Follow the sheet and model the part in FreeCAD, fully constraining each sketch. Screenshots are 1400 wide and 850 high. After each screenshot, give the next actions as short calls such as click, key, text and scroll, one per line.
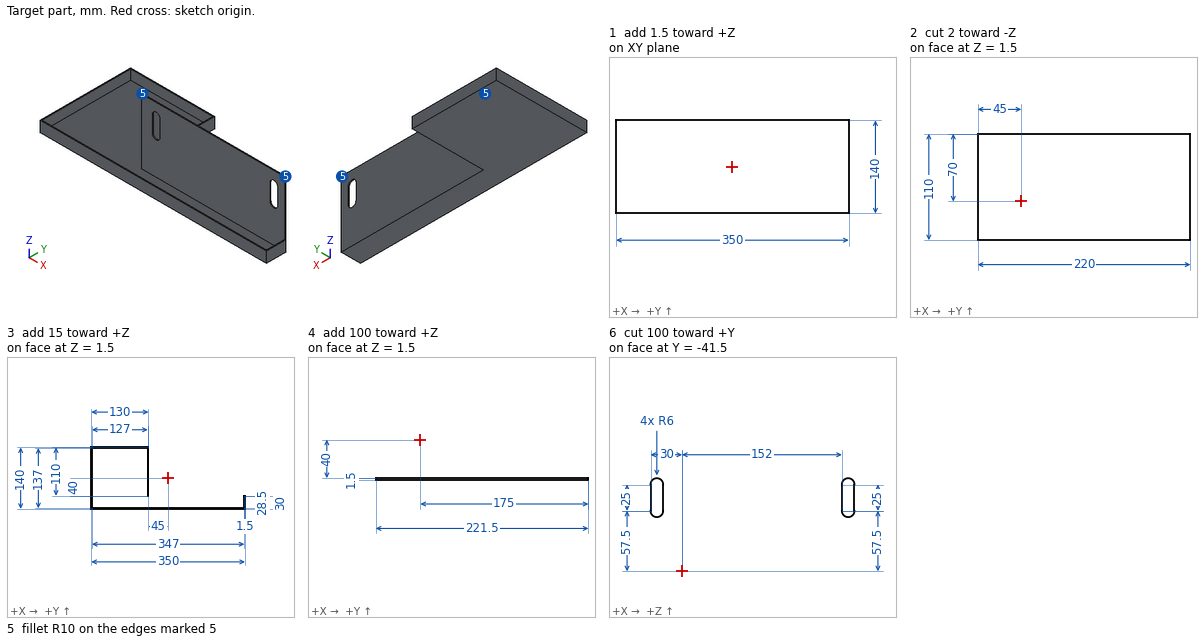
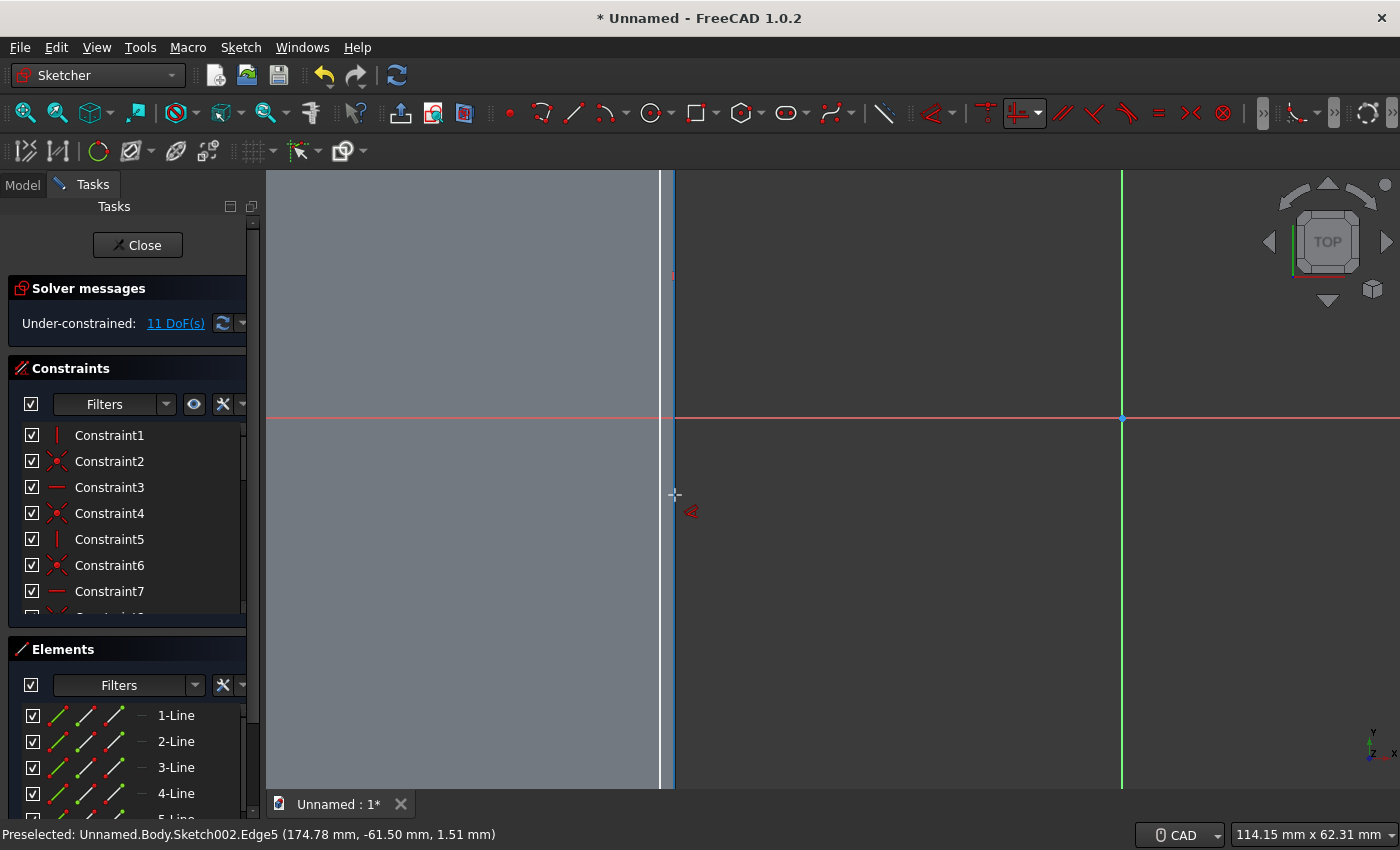
click(674, 491)
click(640, 480)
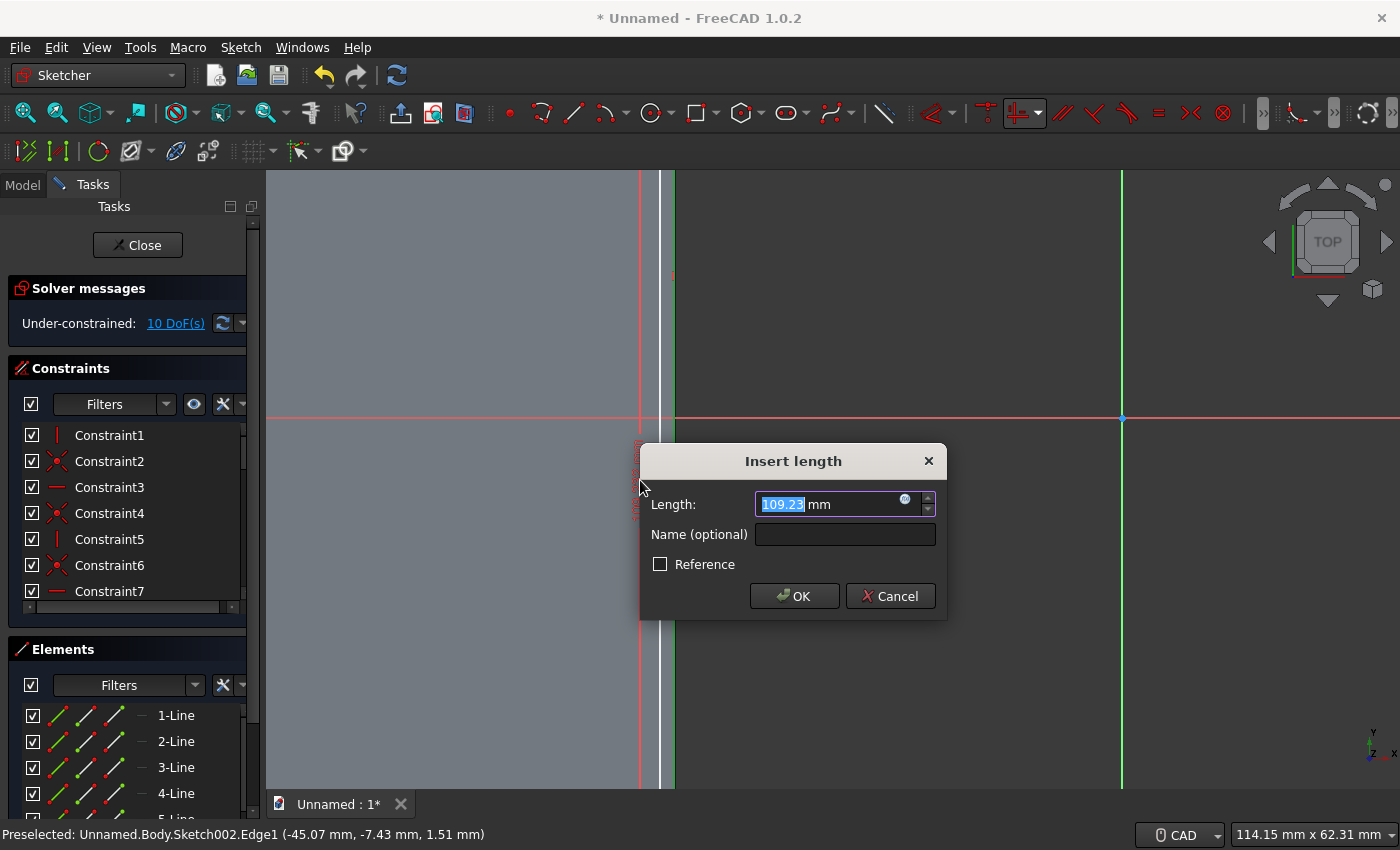
text(110)
key(Return)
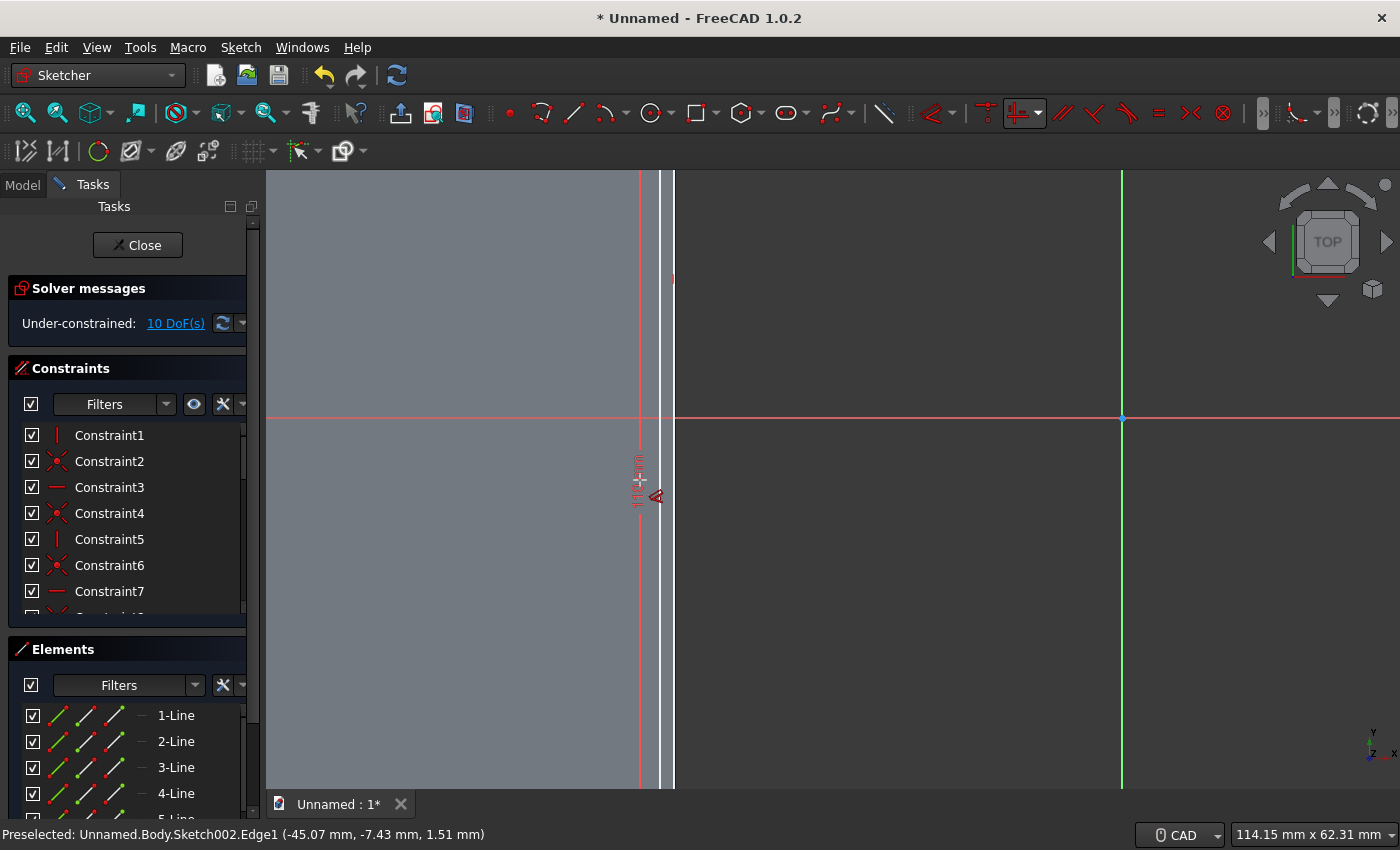
scroll(674, 495, down, 8)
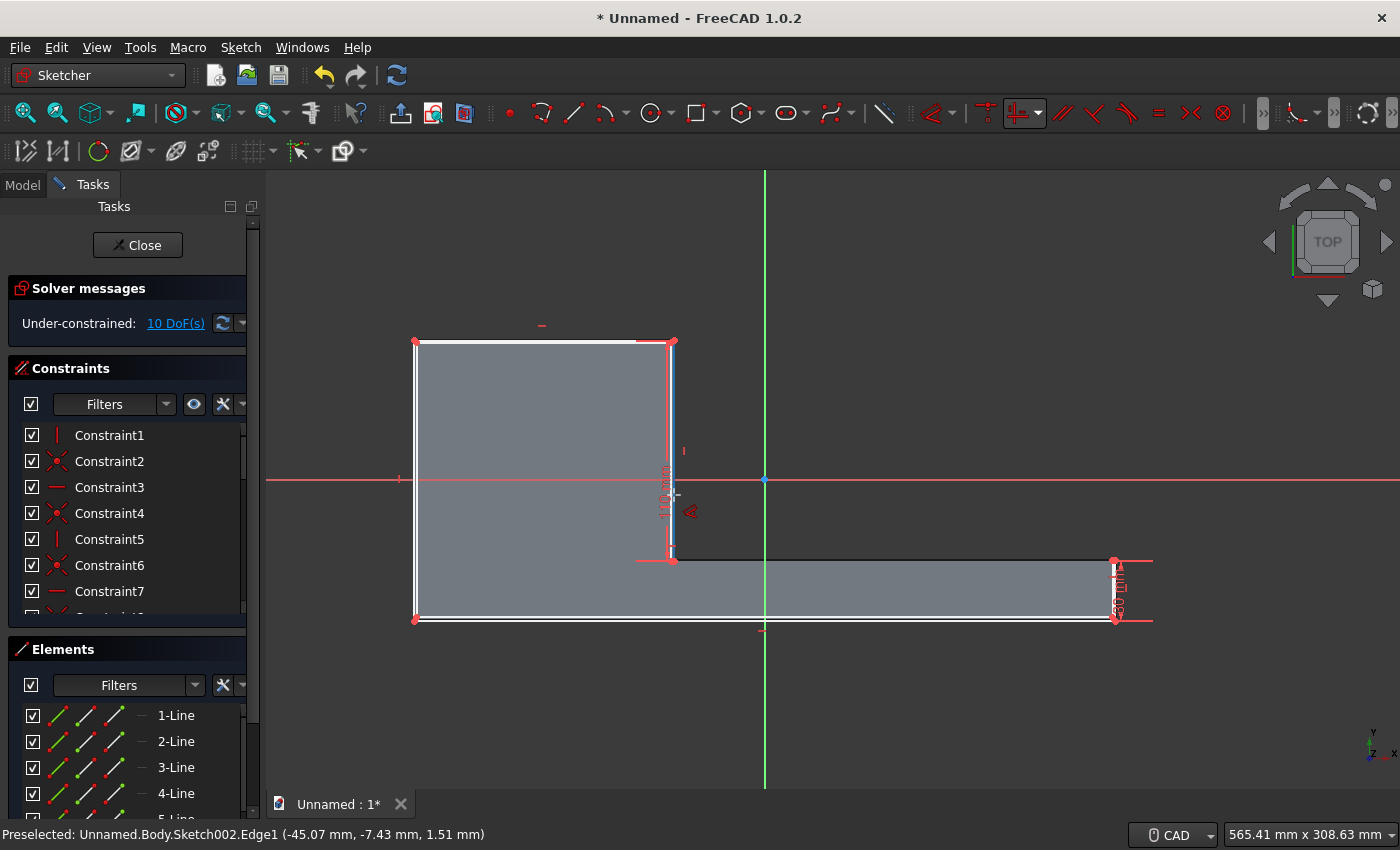
scroll(596, 341, up, 10)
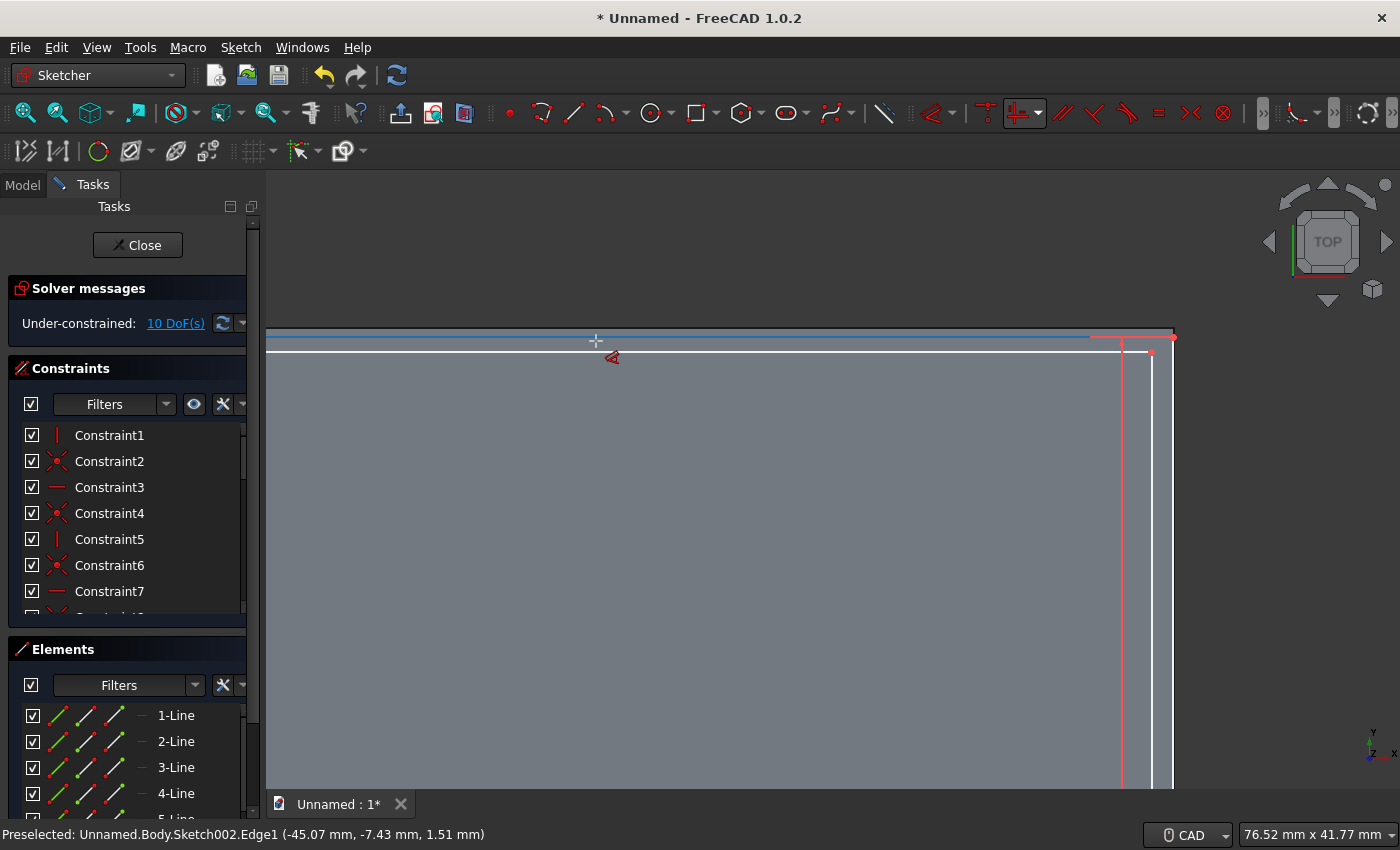
click(596, 337)
click(734, 303)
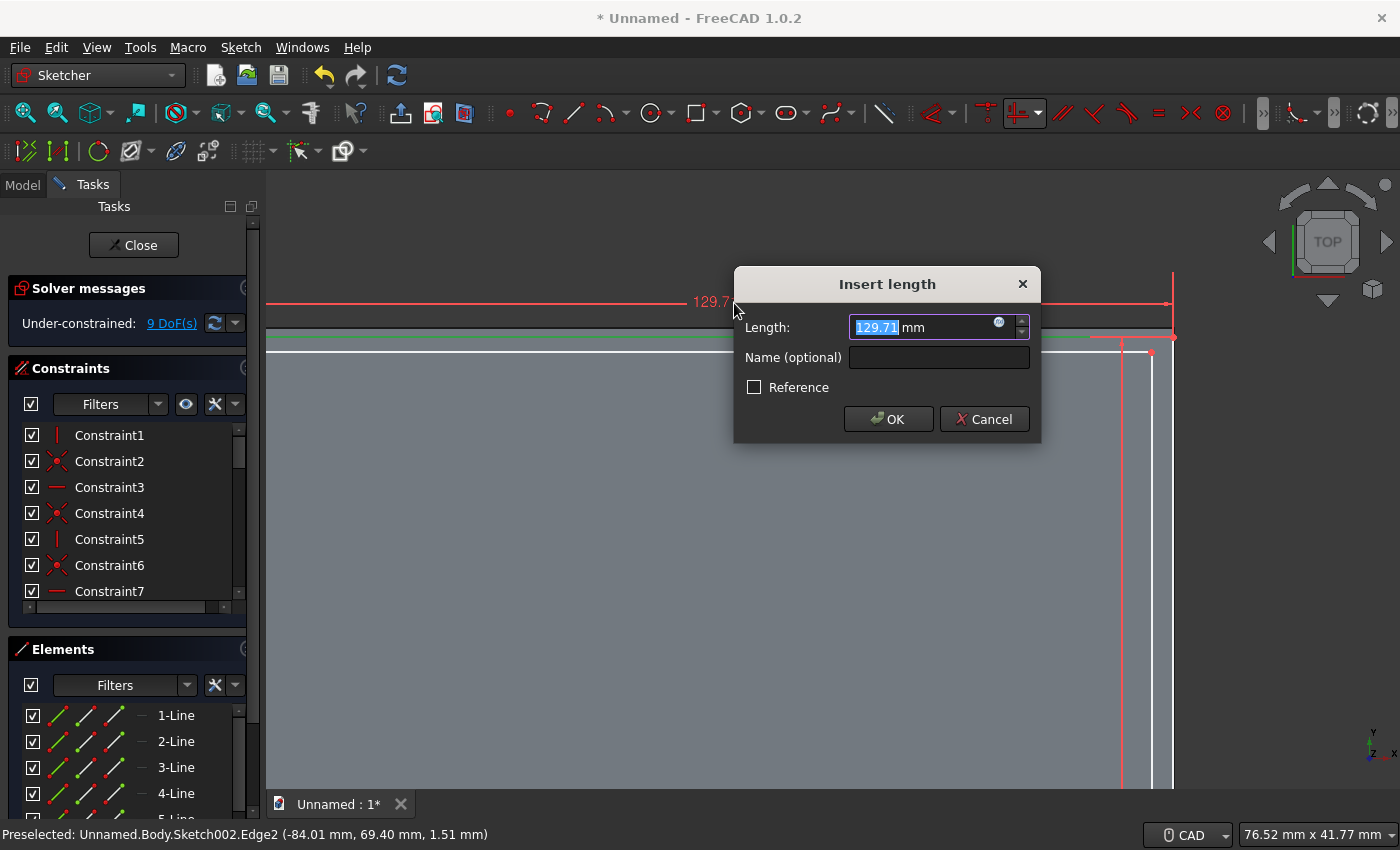
text(130)
key(Return)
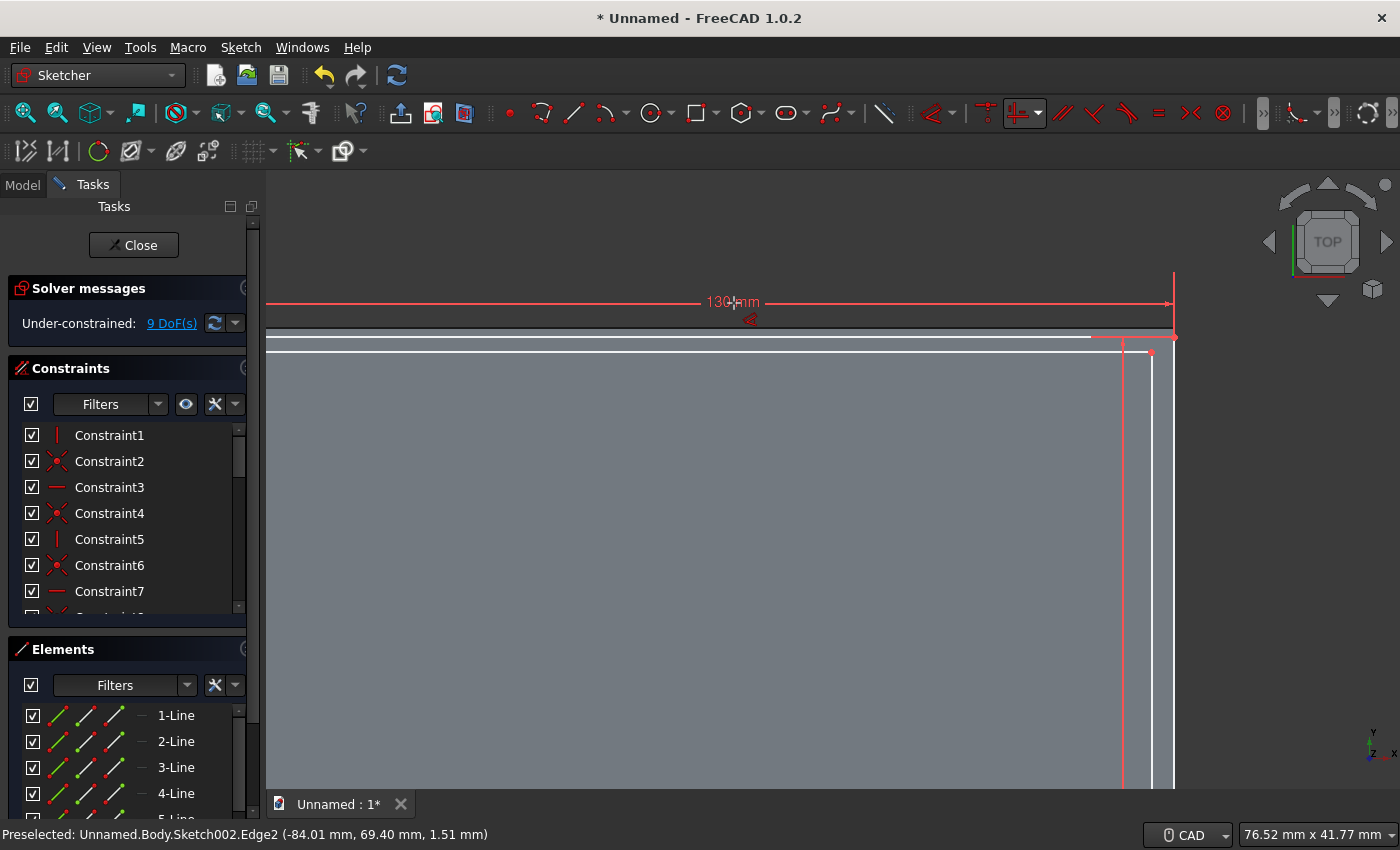
scroll(596, 341, down, 10)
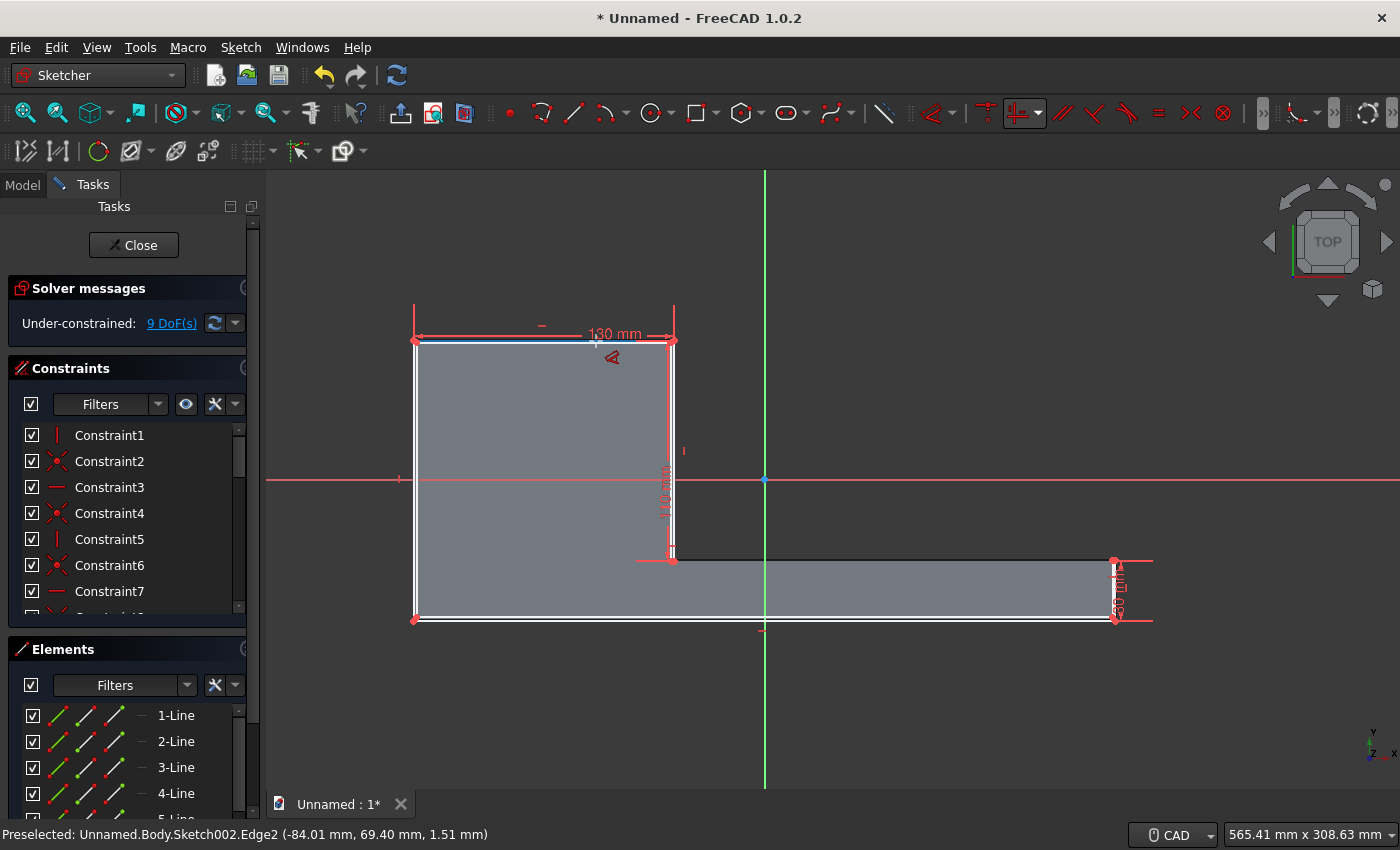
scroll(414, 425, up, 8)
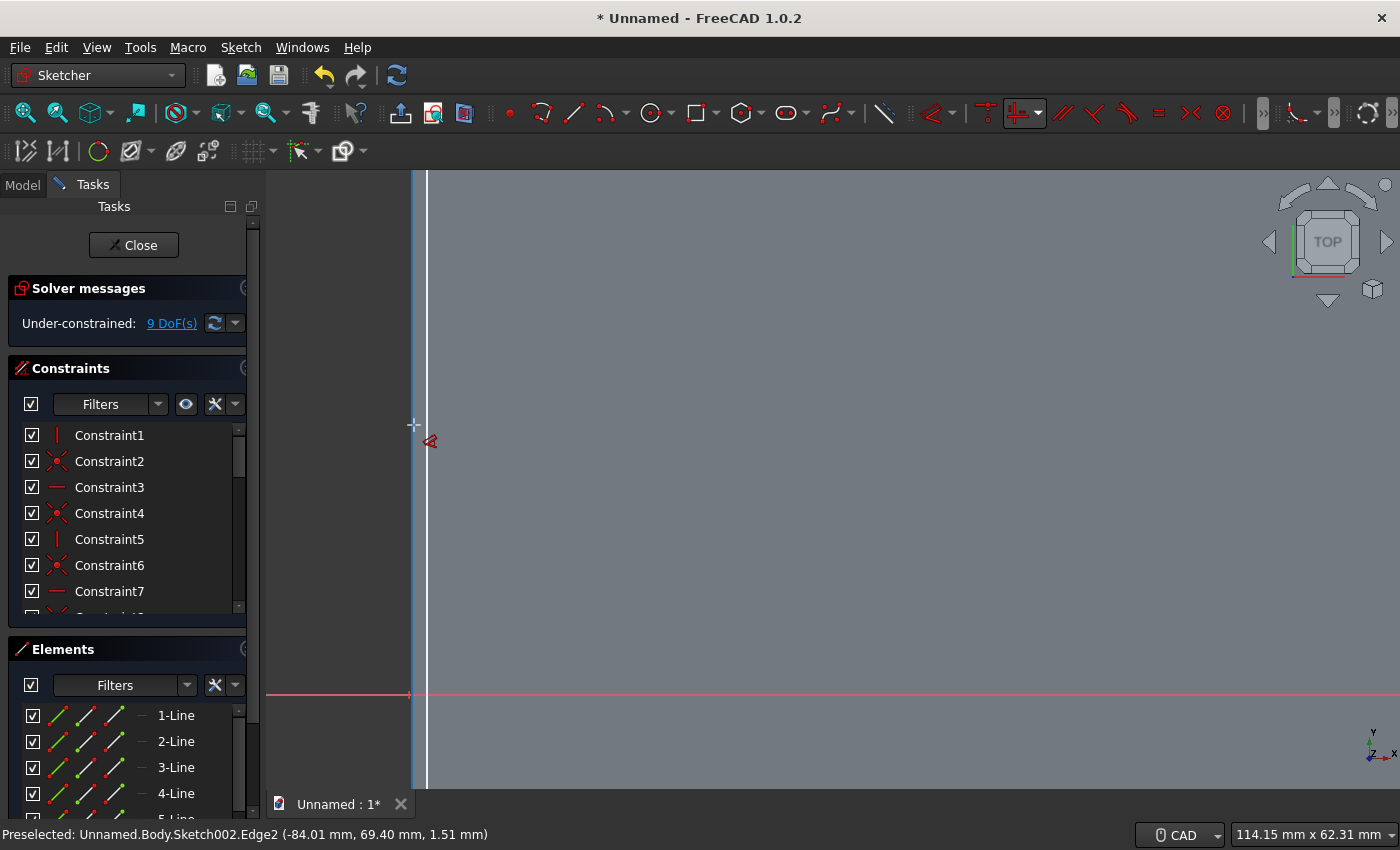
click(412, 423)
click(378, 480)